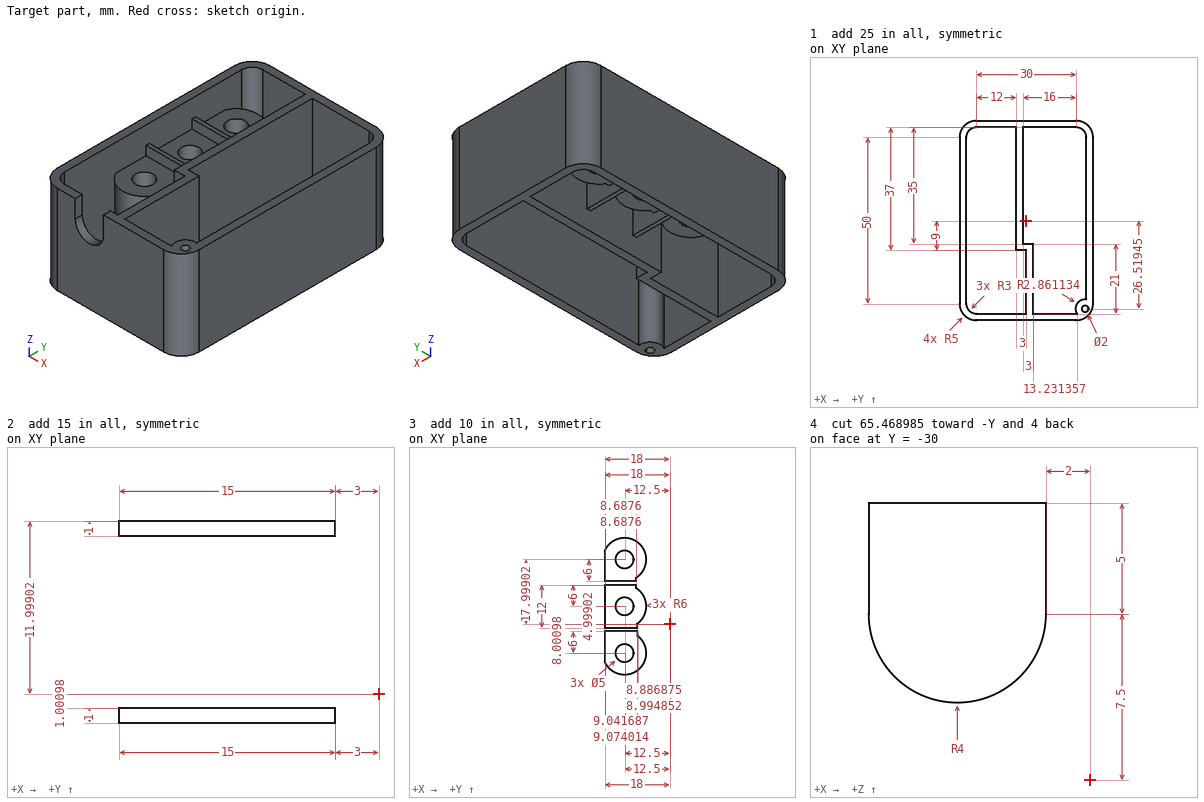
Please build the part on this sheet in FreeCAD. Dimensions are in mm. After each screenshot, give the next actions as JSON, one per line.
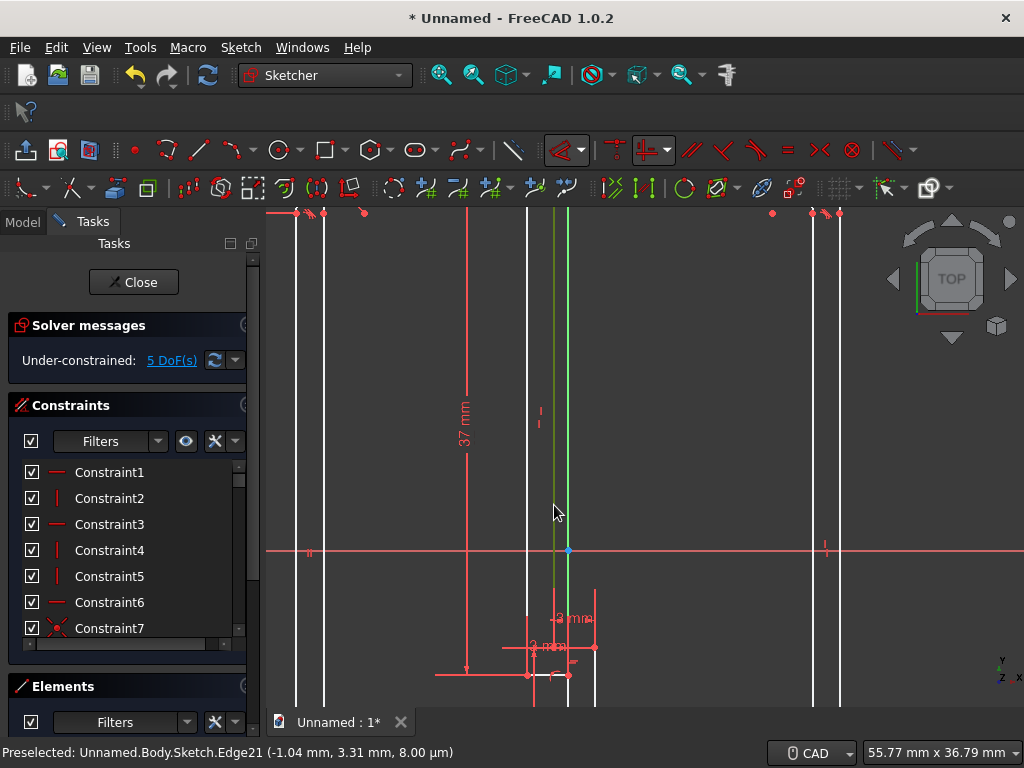
{"action": "left_click", "coordinate": [584, 150]}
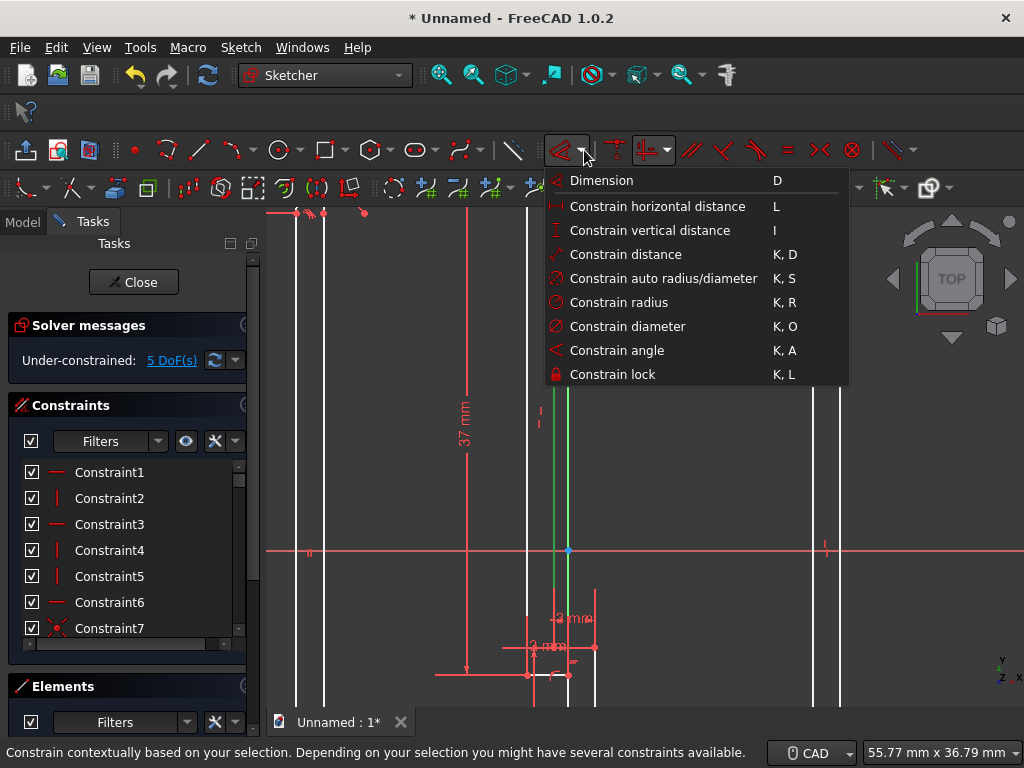
{"action": "left_click", "coordinate": [697, 230]}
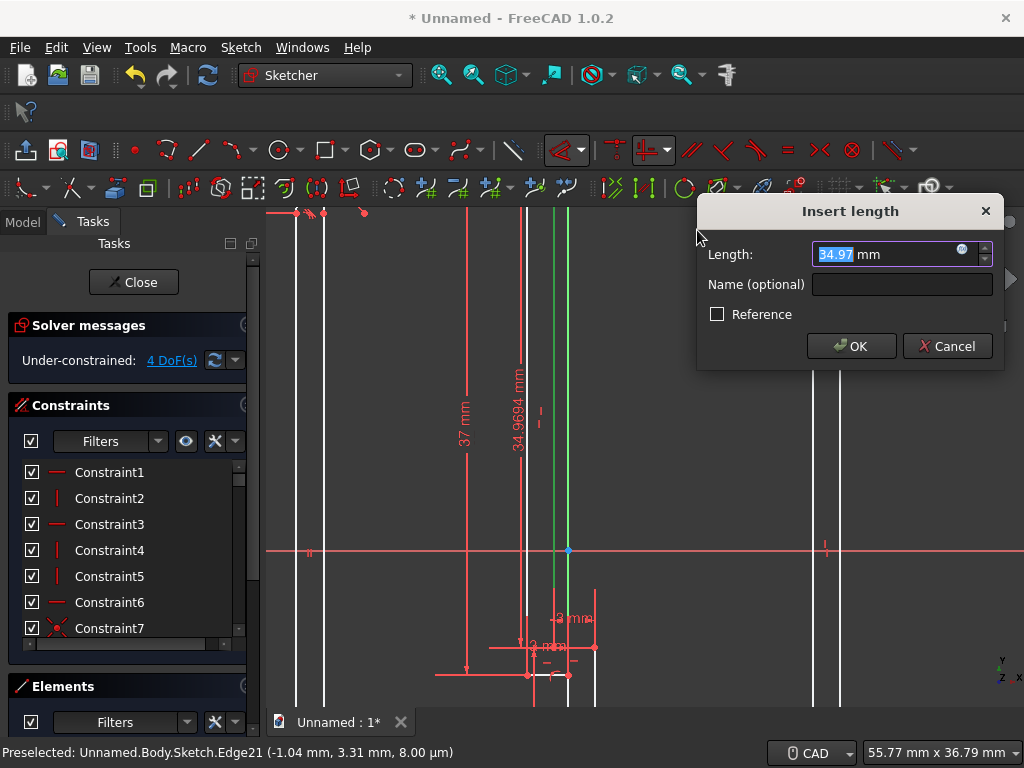
{"action": "type", "text": "35"}
{"action": "key", "text": "Return"}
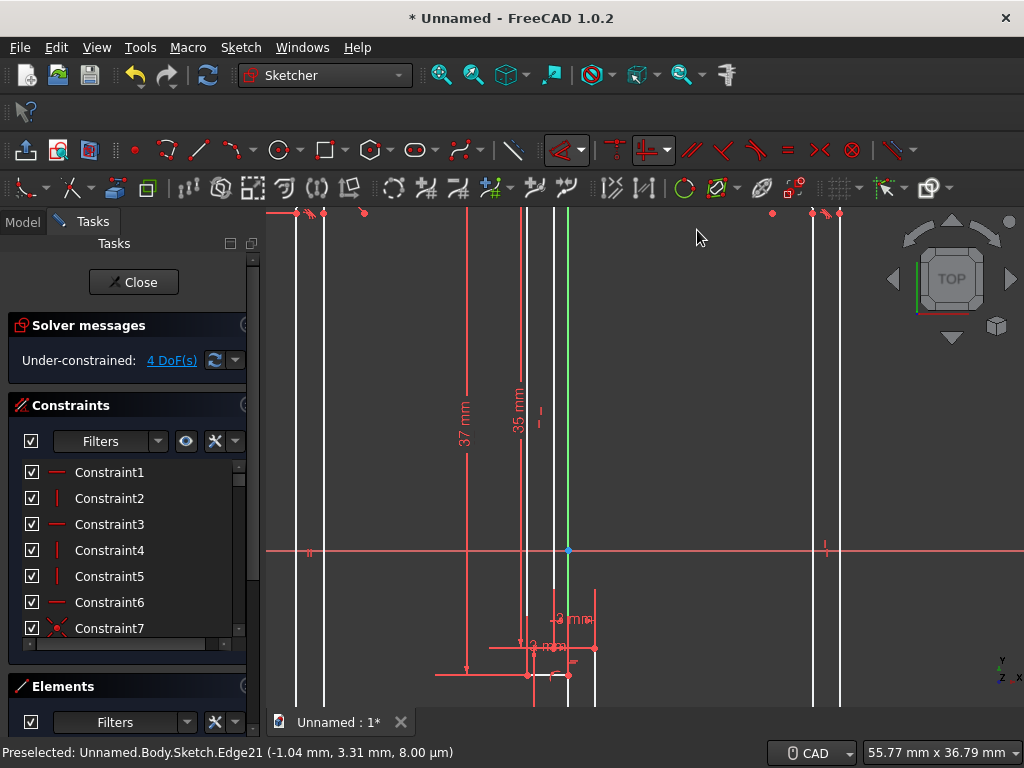
{"action": "scroll", "coordinate": [581, 402], "scroll_direction": "down", "scroll_amount": 5}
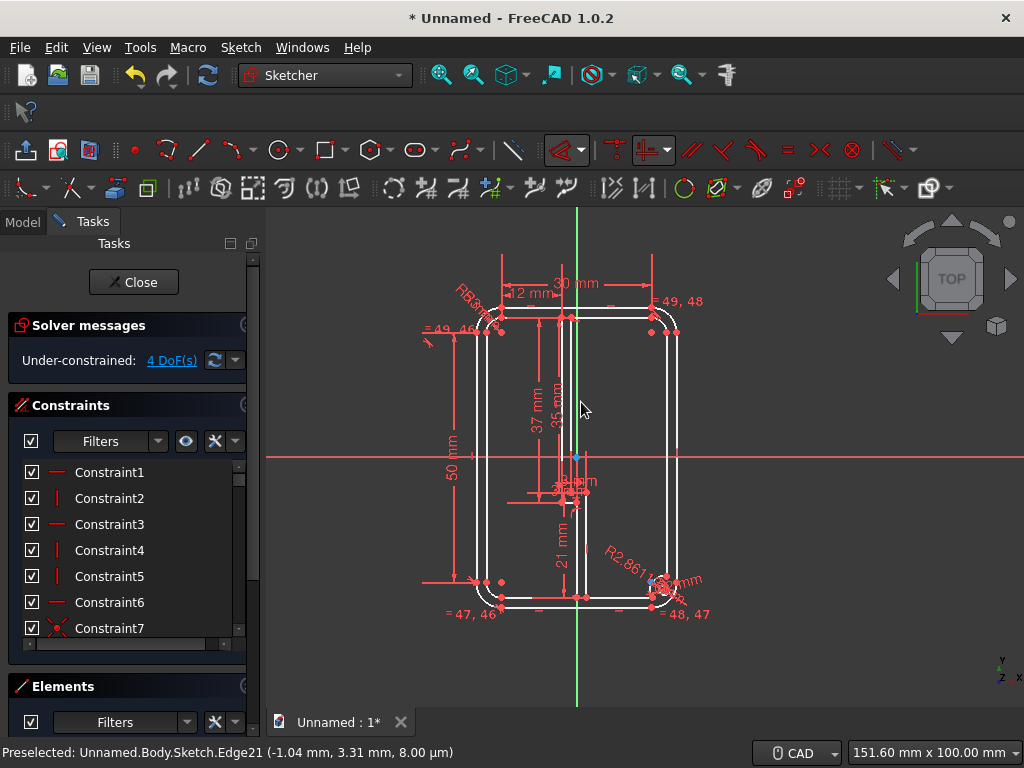
{"action": "scroll", "coordinate": [595, 318], "scroll_direction": "up", "scroll_amount": 2}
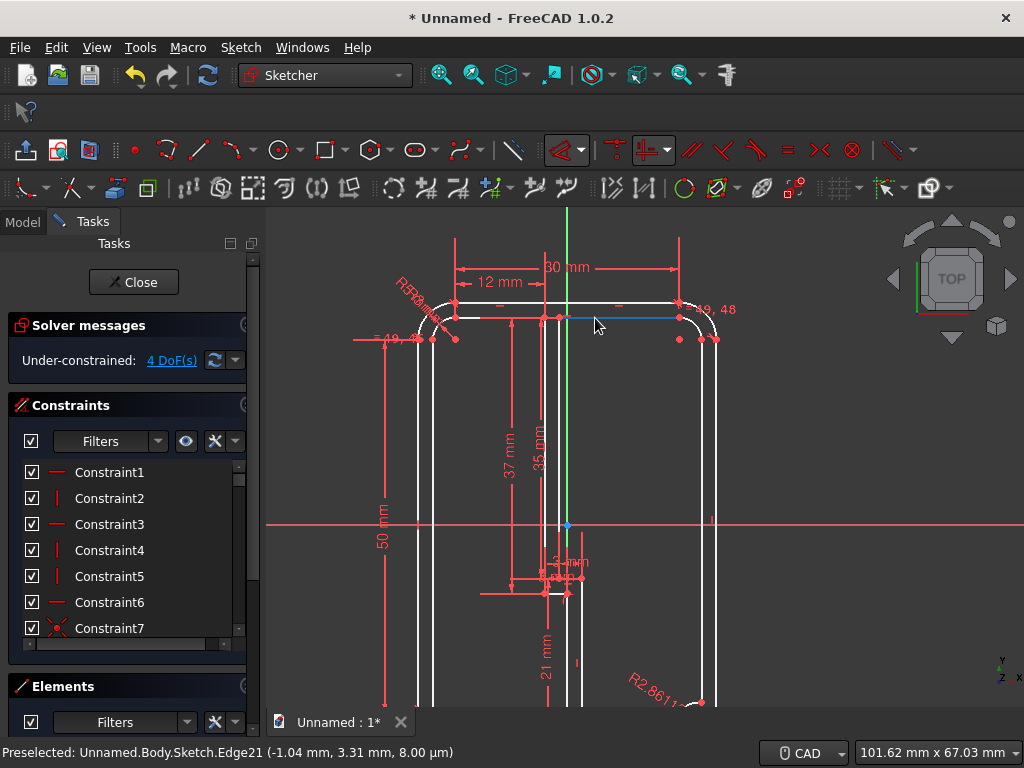
{"action": "left_click", "coordinate": [595, 318]}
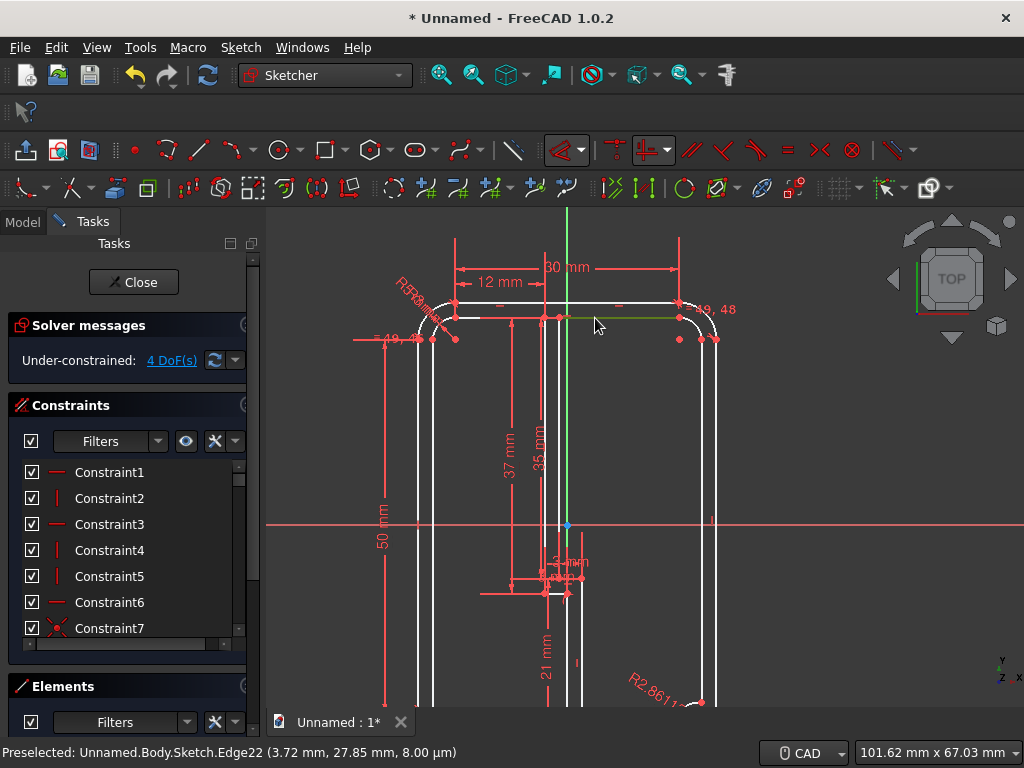
{"action": "left_click", "coordinate": [584, 150]}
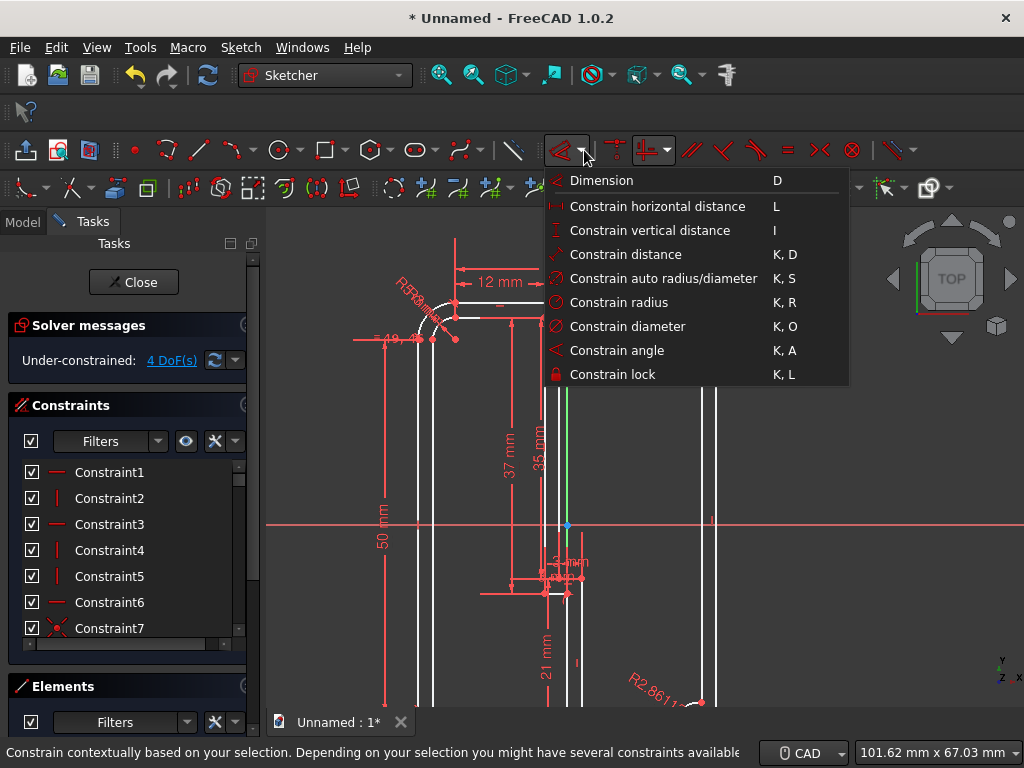
{"action": "left_click", "coordinate": [697, 206]}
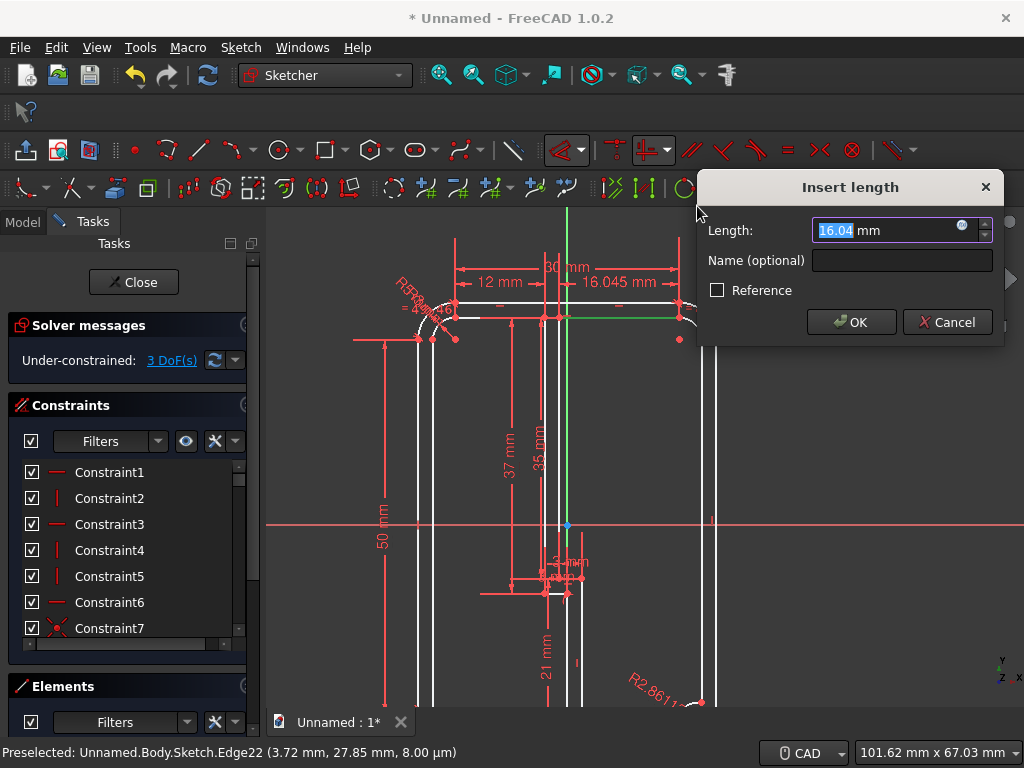
{"action": "type", "text": "16"}
{"action": "key", "text": "Return"}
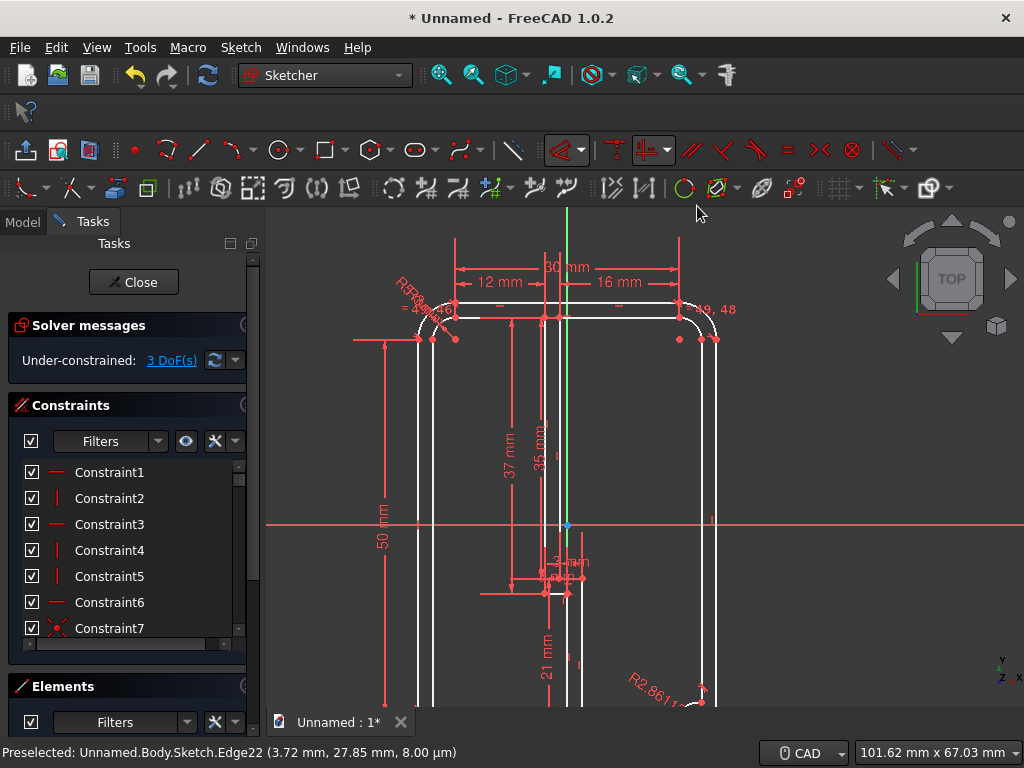
{"action": "left_click", "coordinate": [545, 594]}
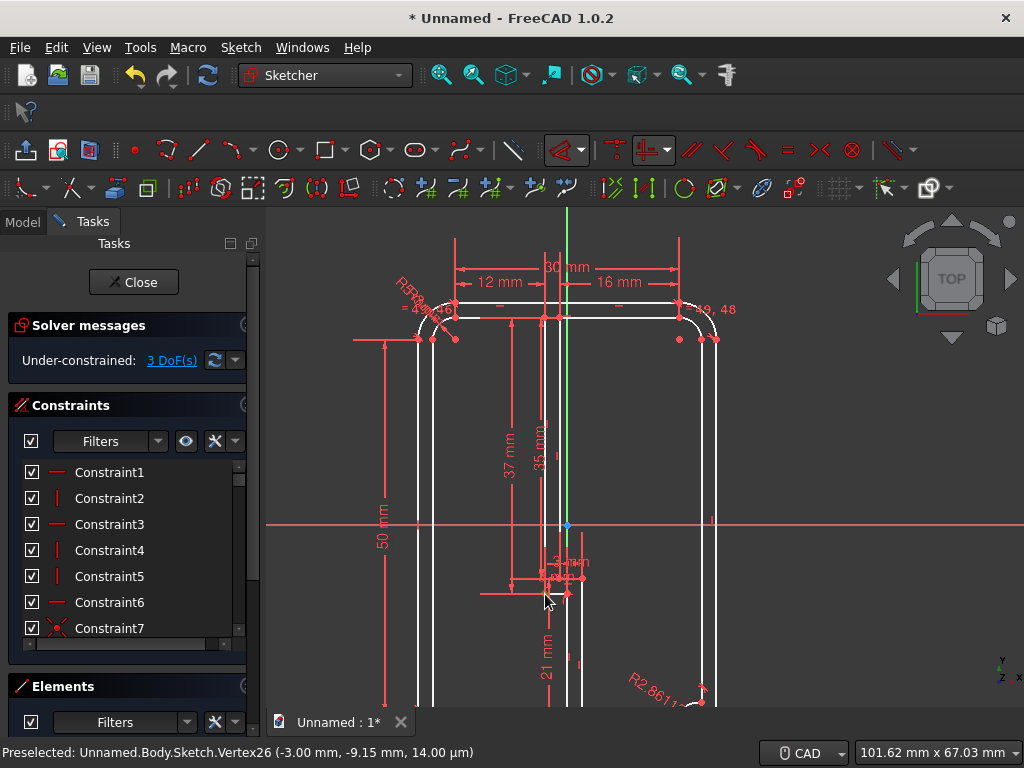
{"action": "left_click", "coordinate": [584, 150]}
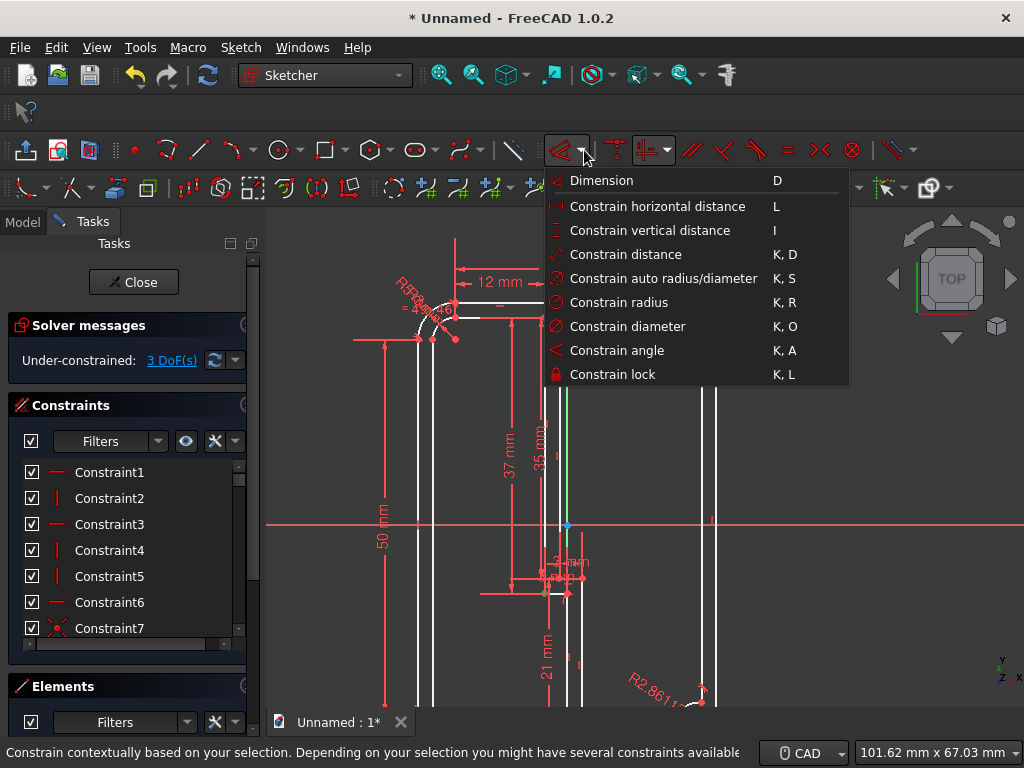
{"action": "left_click", "coordinate": [697, 230]}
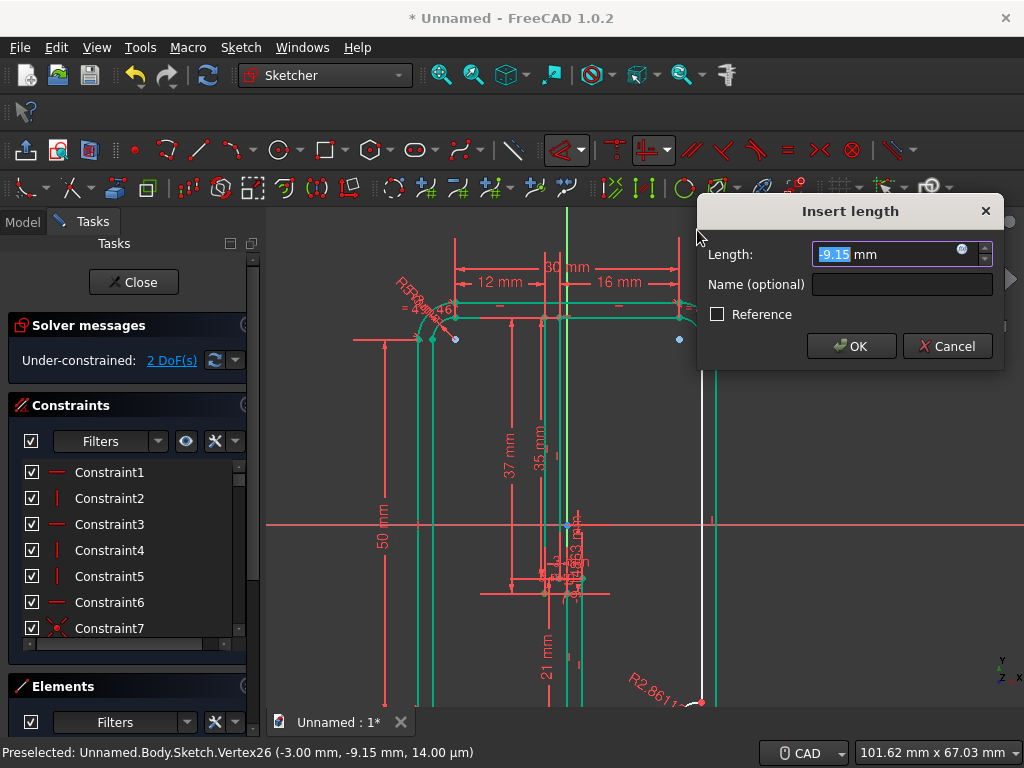
{"action": "type", "text": "-9"}
{"action": "key", "text": "Return"}